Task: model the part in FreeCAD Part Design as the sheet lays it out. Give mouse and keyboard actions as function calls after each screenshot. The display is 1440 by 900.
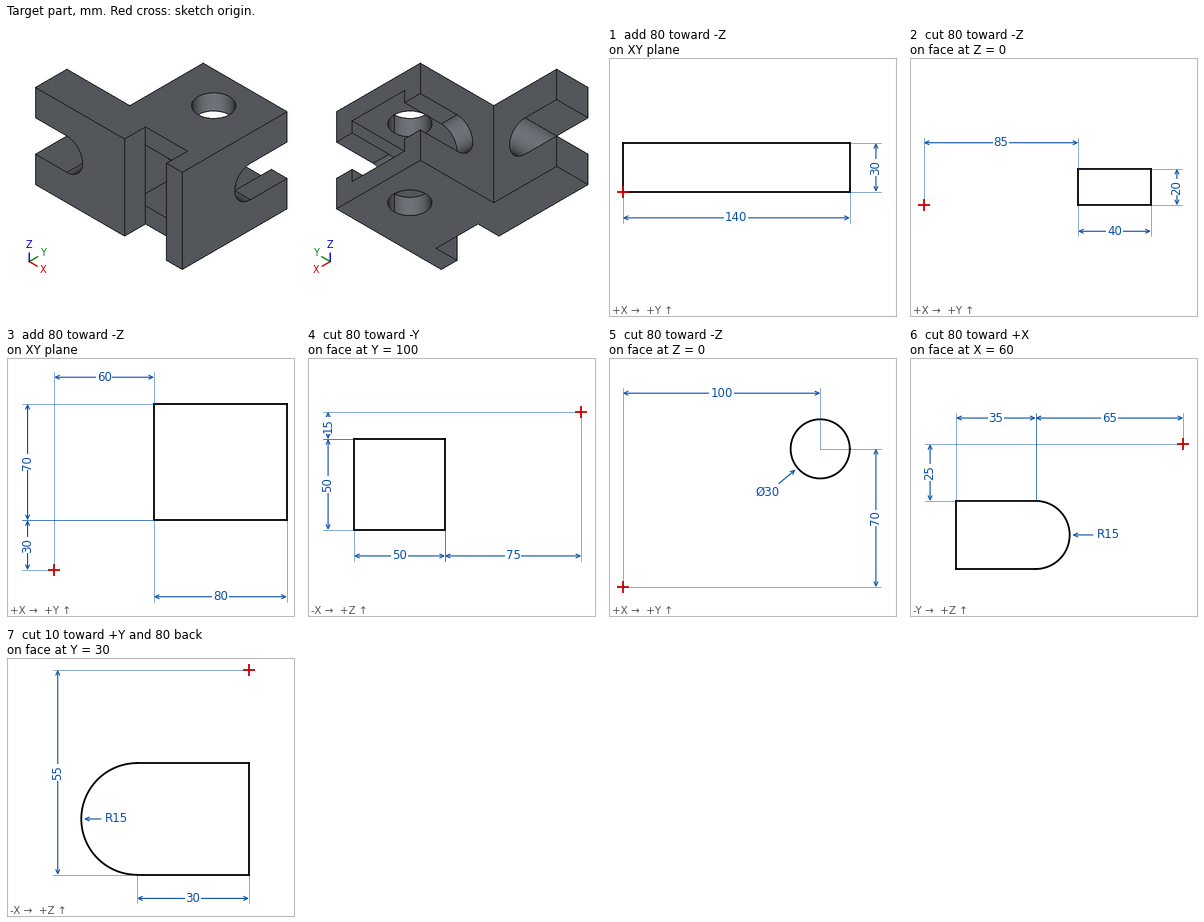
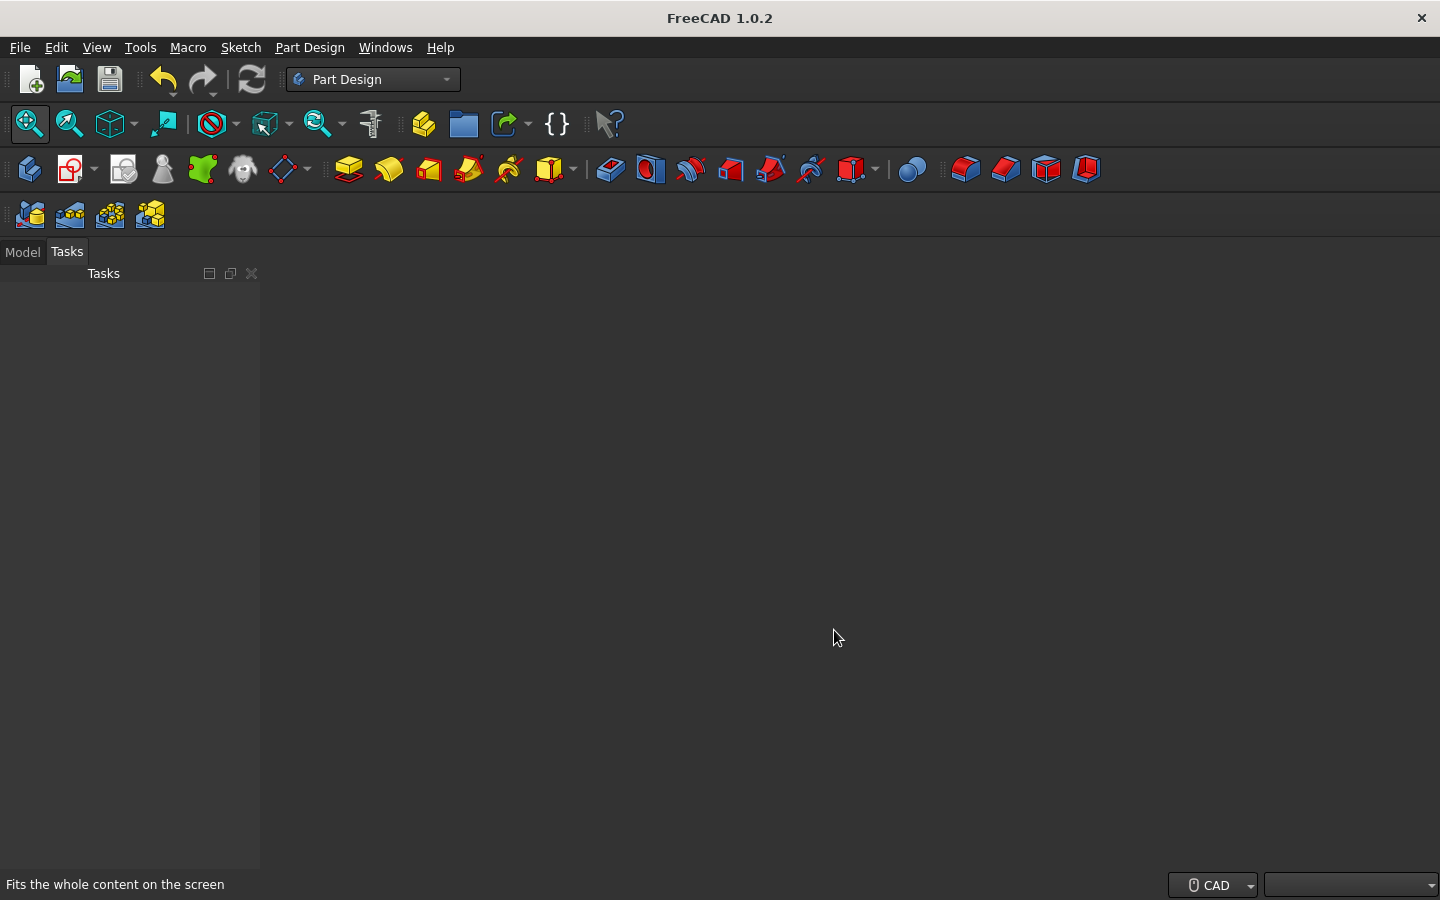
key(ctrl+n)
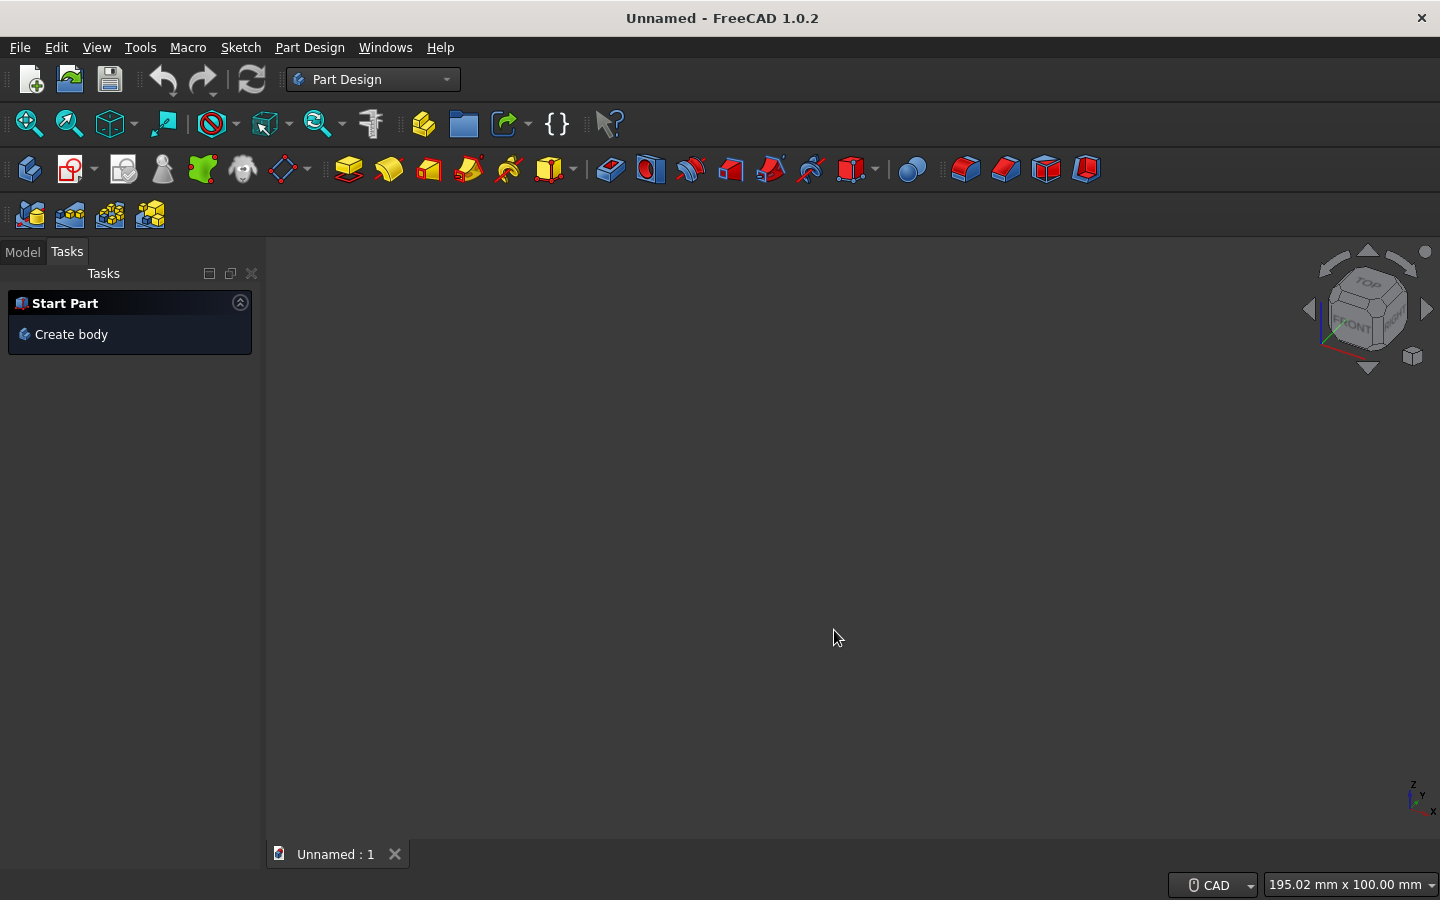
click(70, 170)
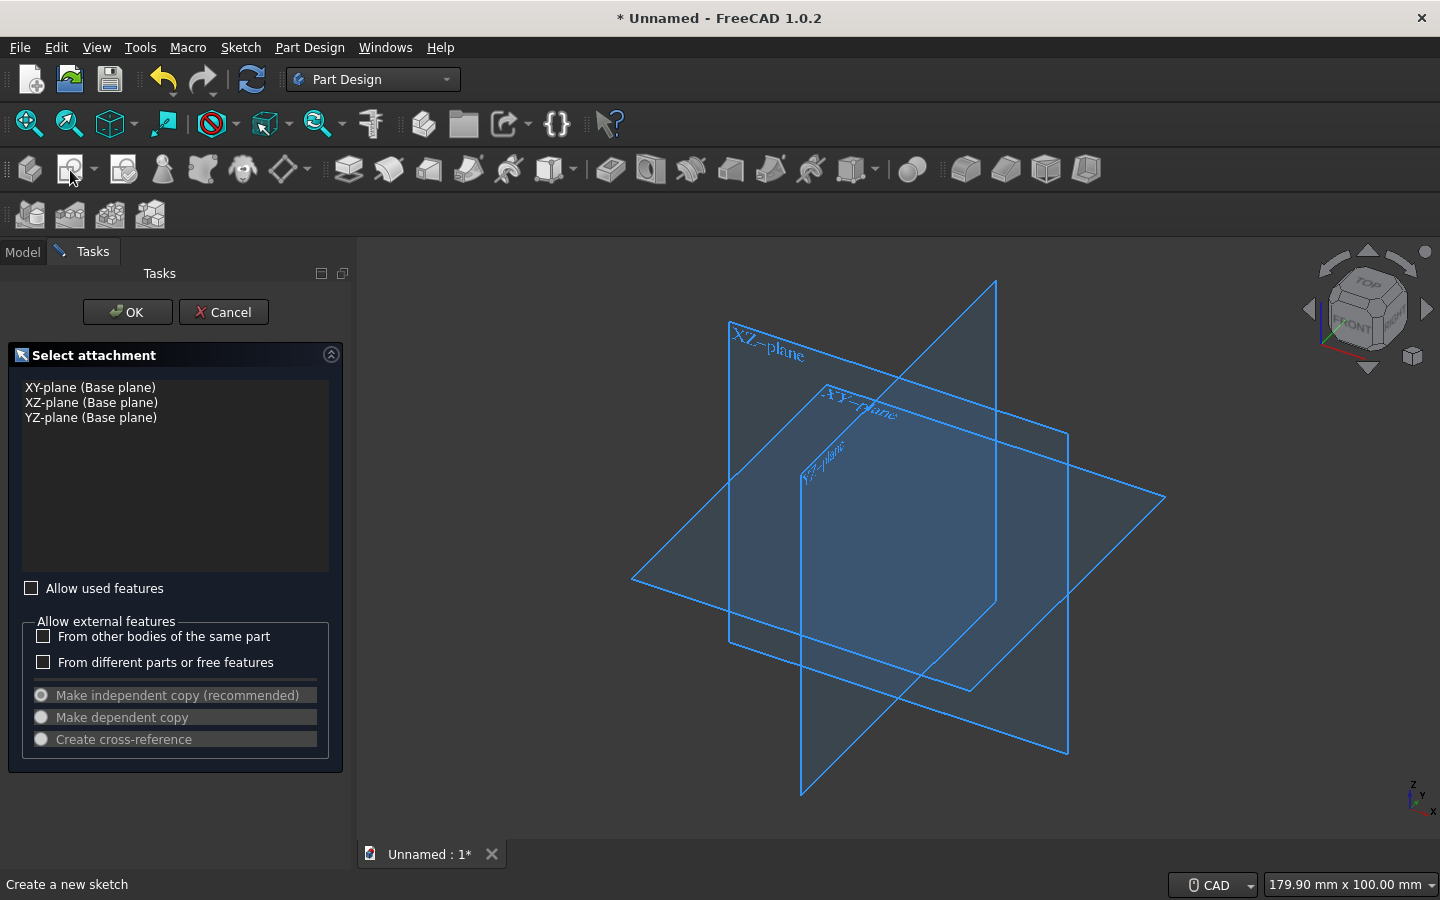
click(82, 388)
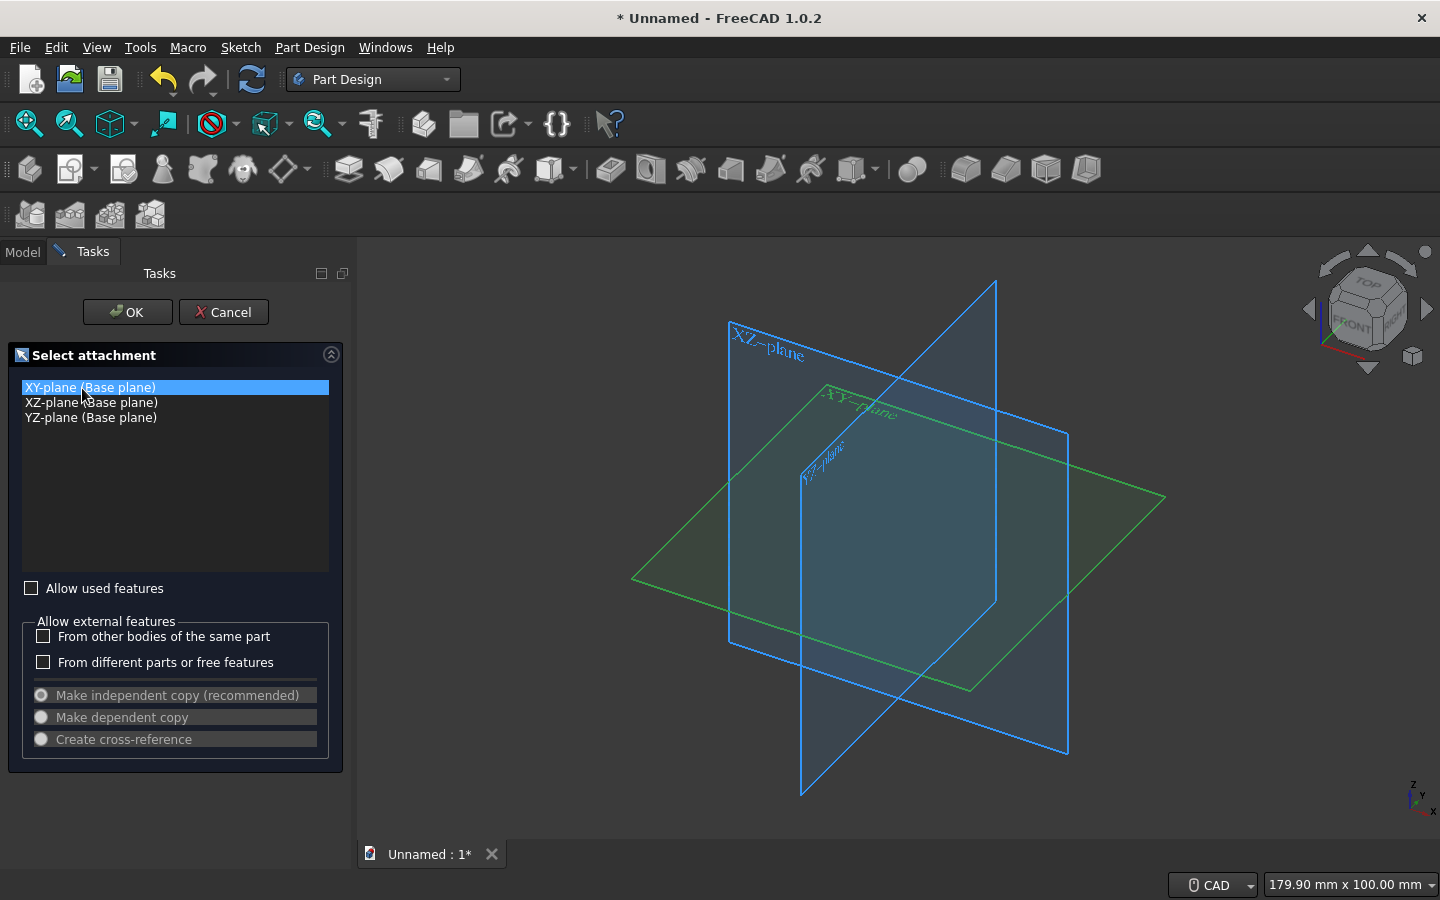
click(128, 312)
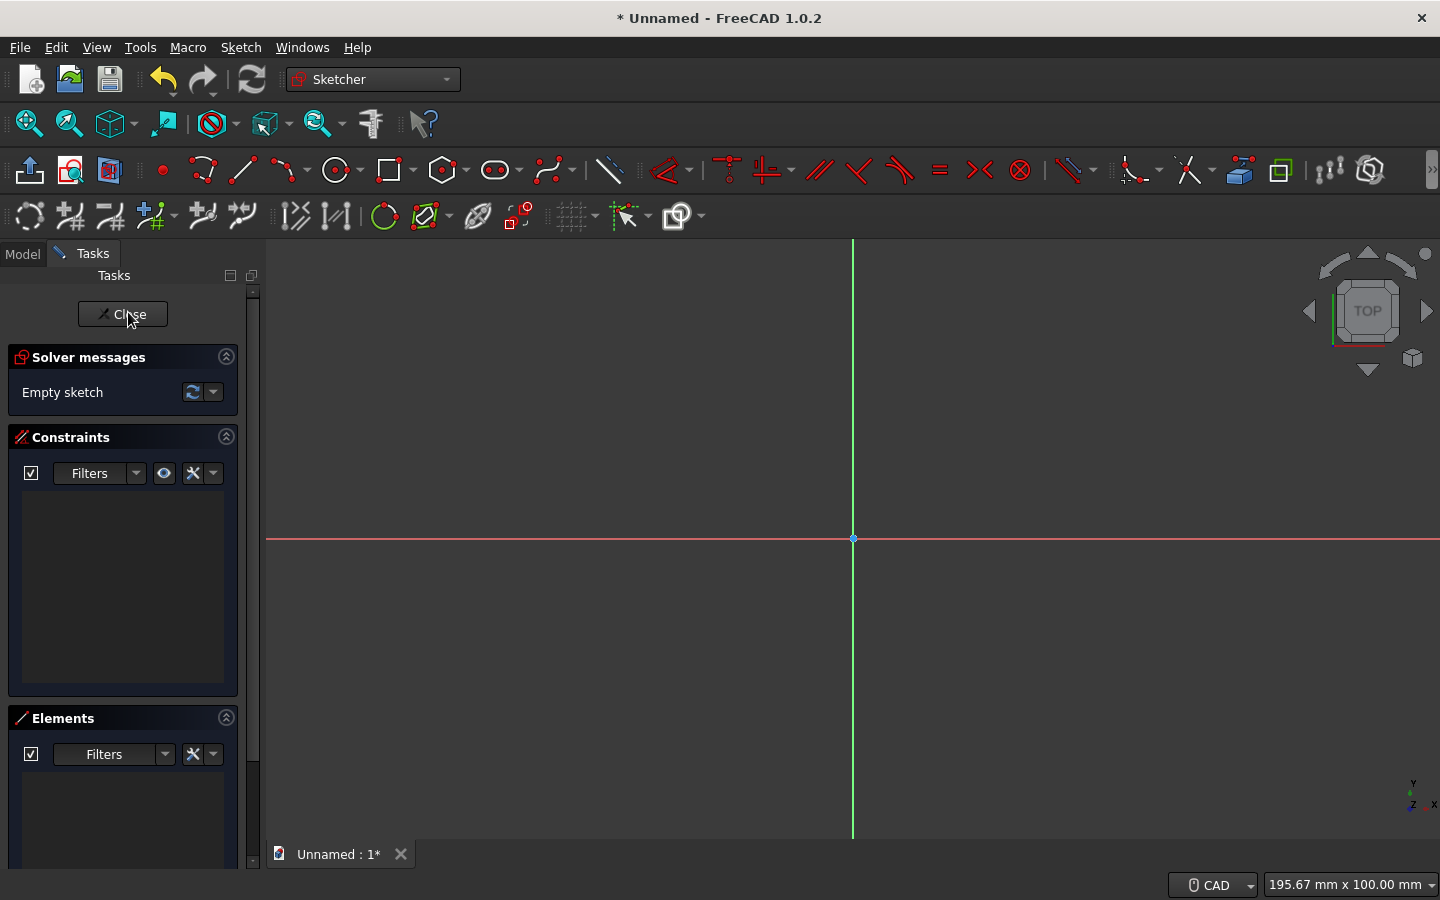
scroll(294, 722, down, 2)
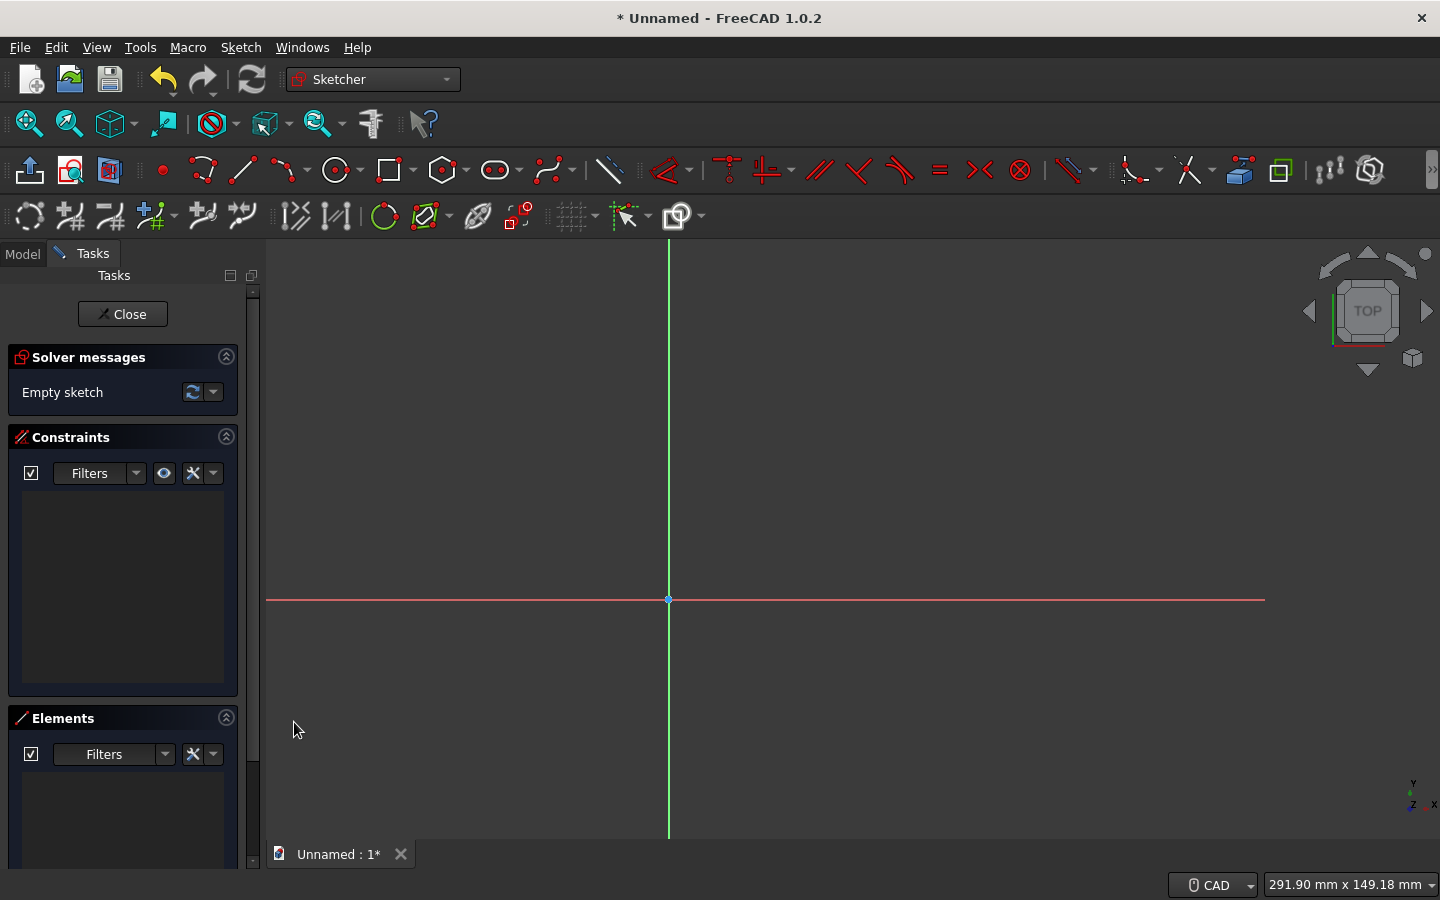
key(g)
key(r)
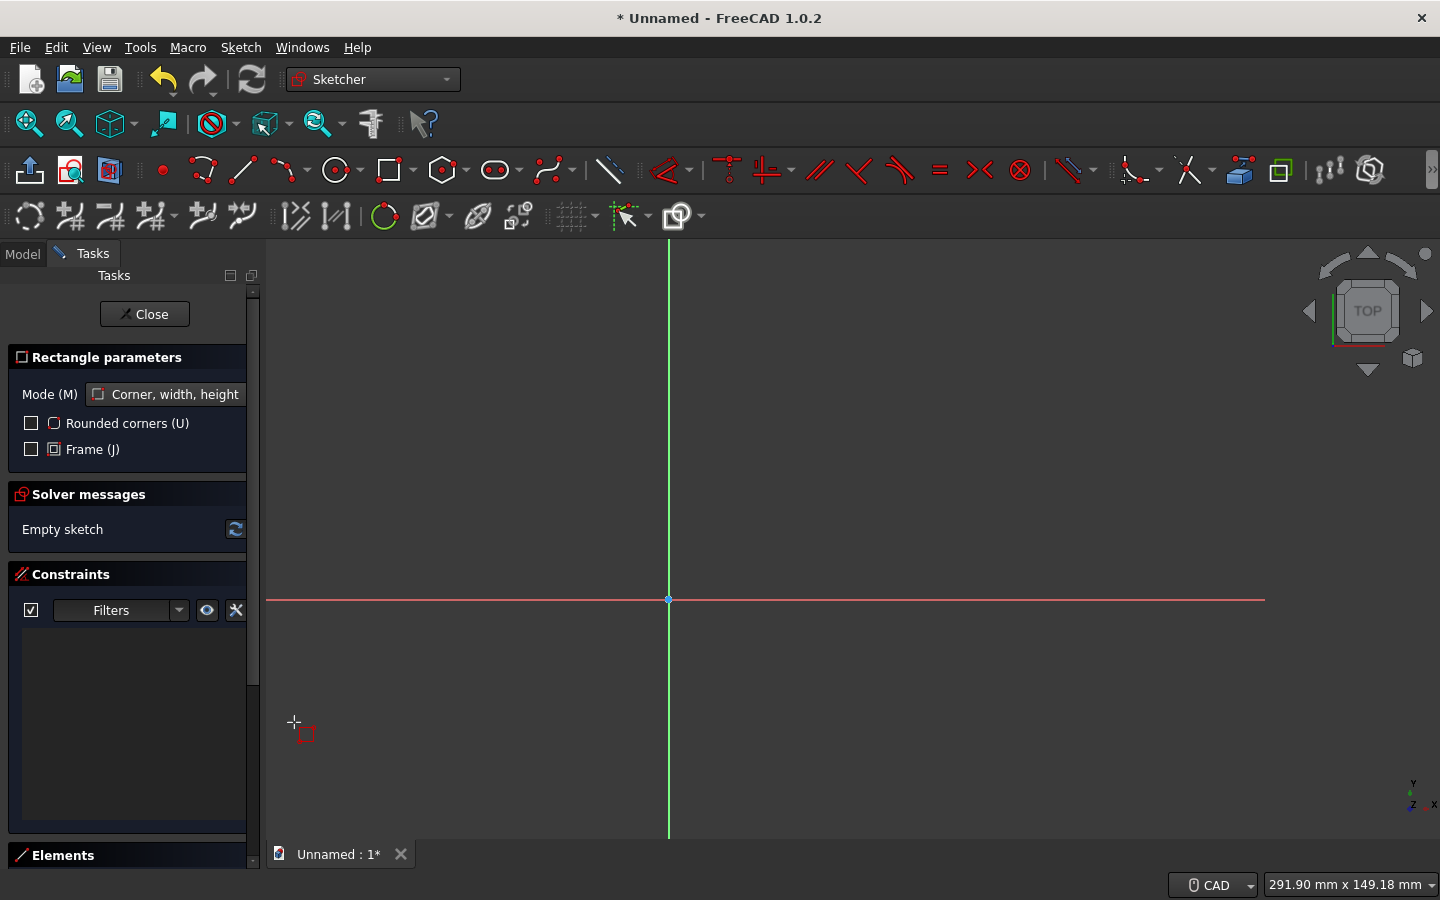
click(669, 600)
click(1232, 479)
key(Escape)